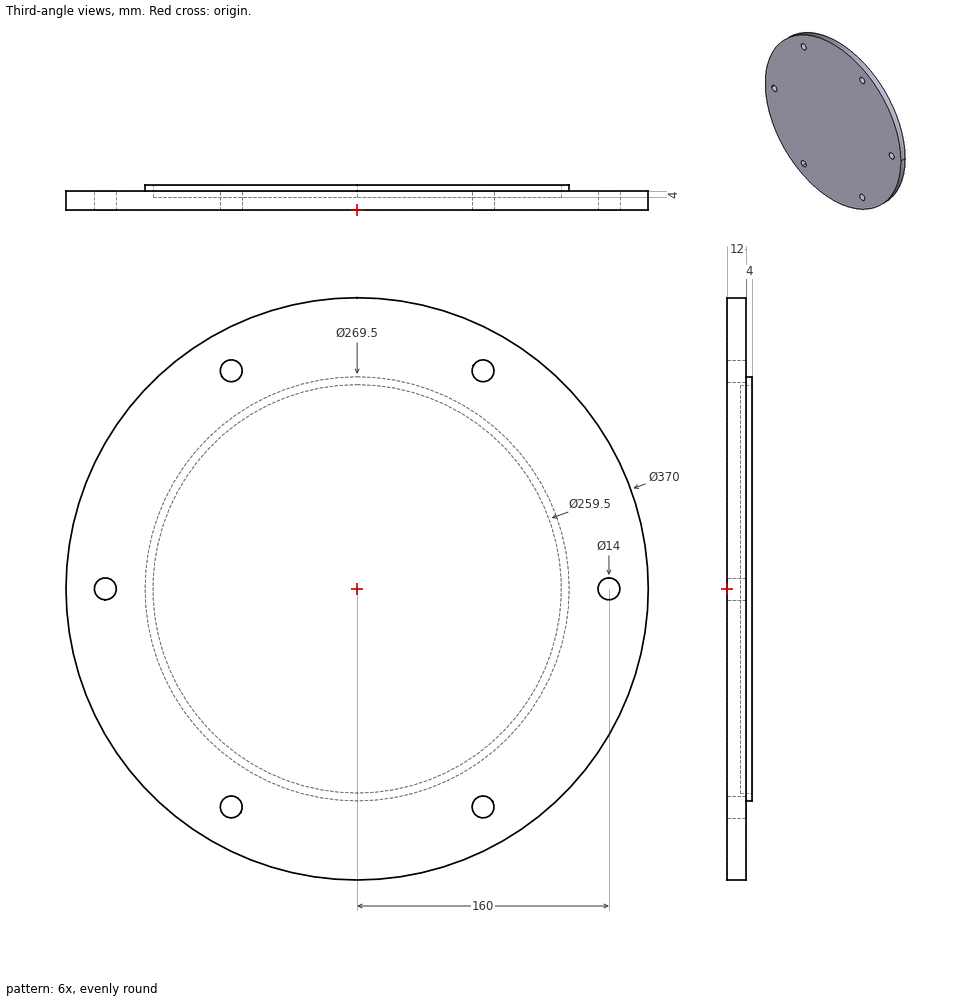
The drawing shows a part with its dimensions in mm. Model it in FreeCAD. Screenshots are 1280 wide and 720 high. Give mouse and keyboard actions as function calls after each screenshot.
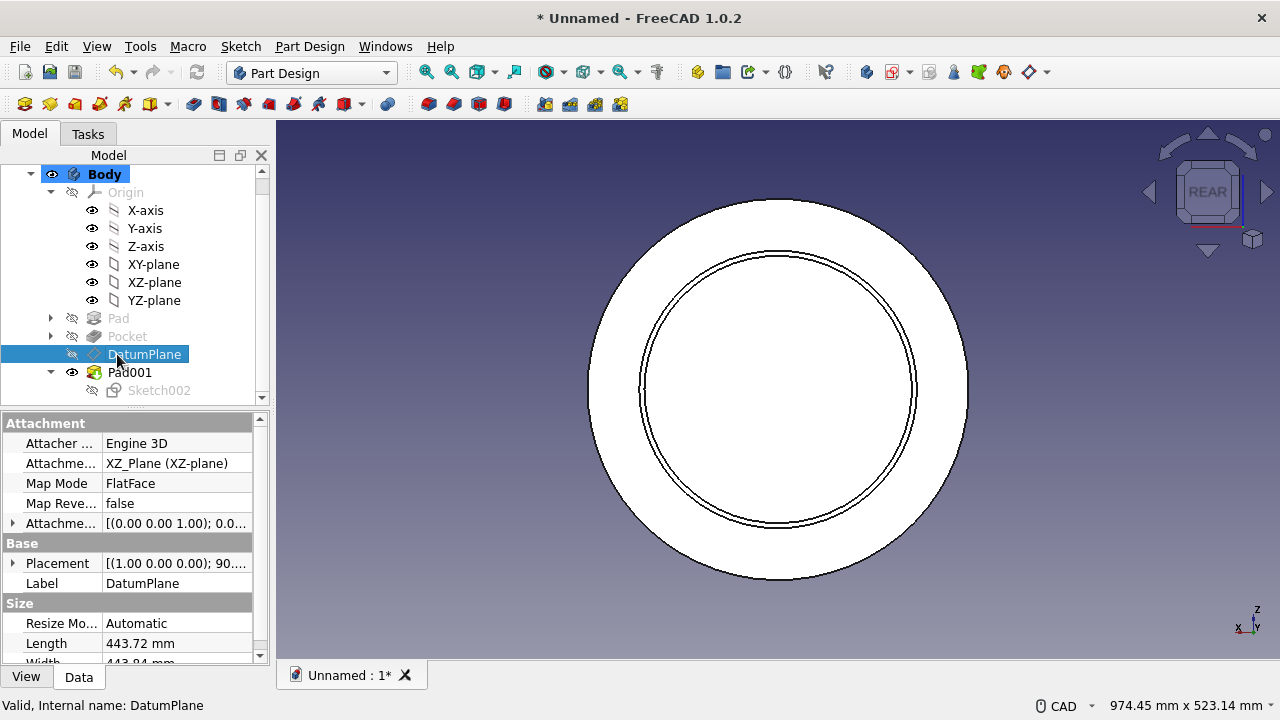
click(778, 552)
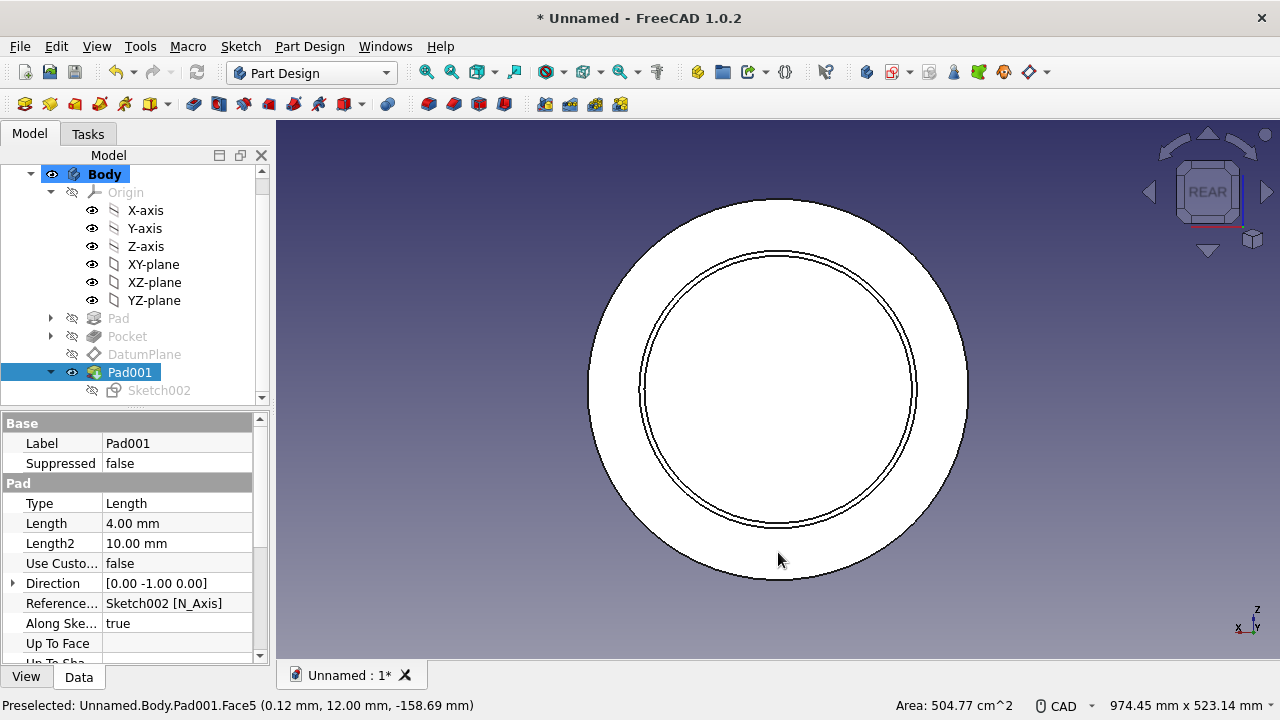
click(892, 72)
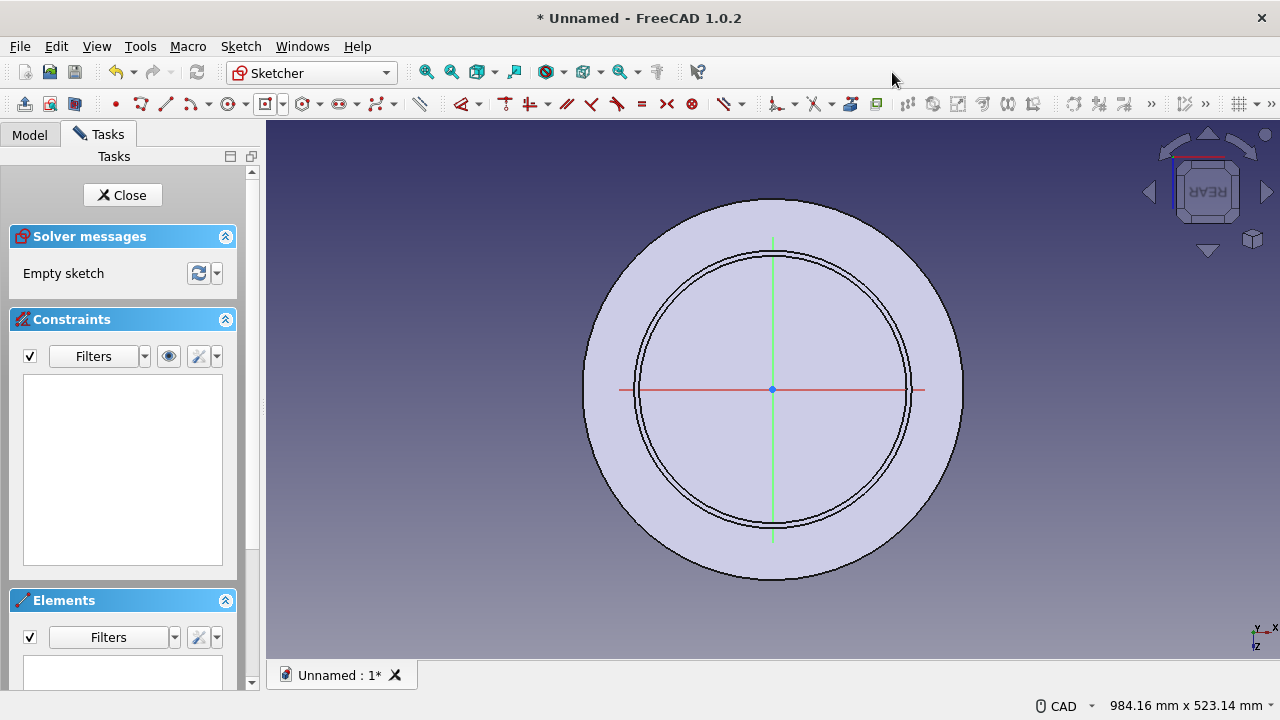
click(75, 104)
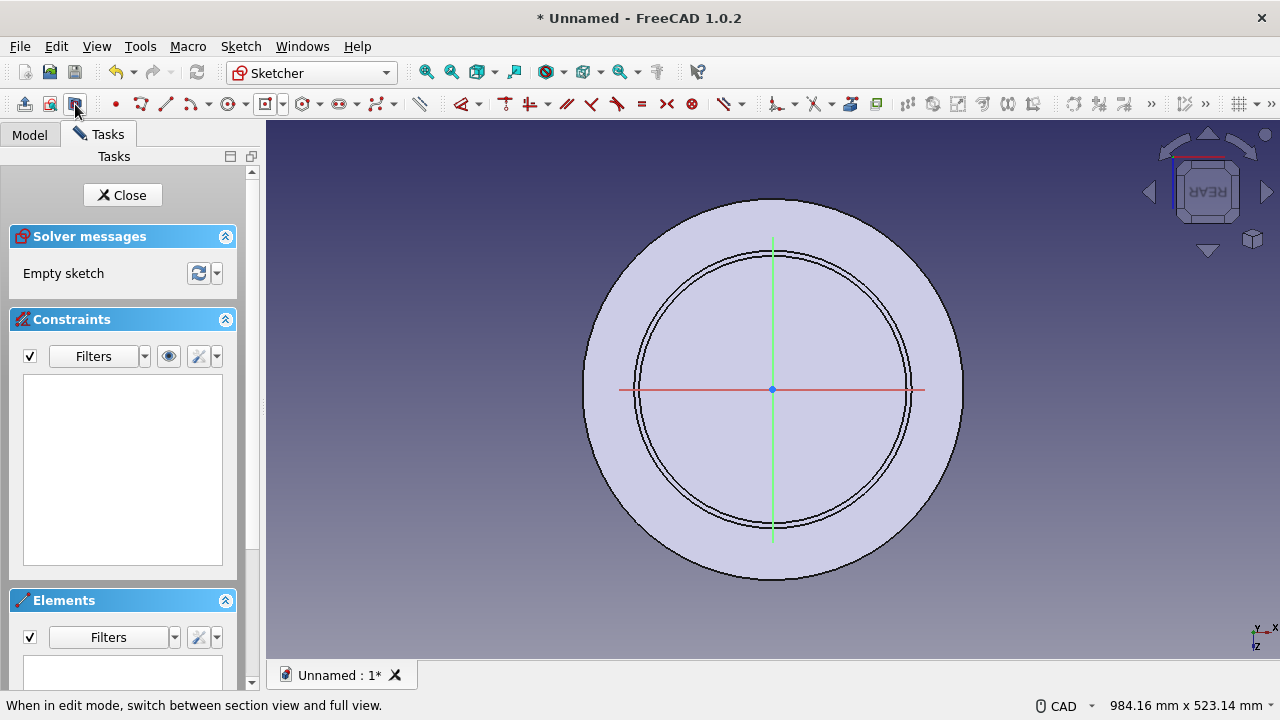
scroll(950, 389, up, 15)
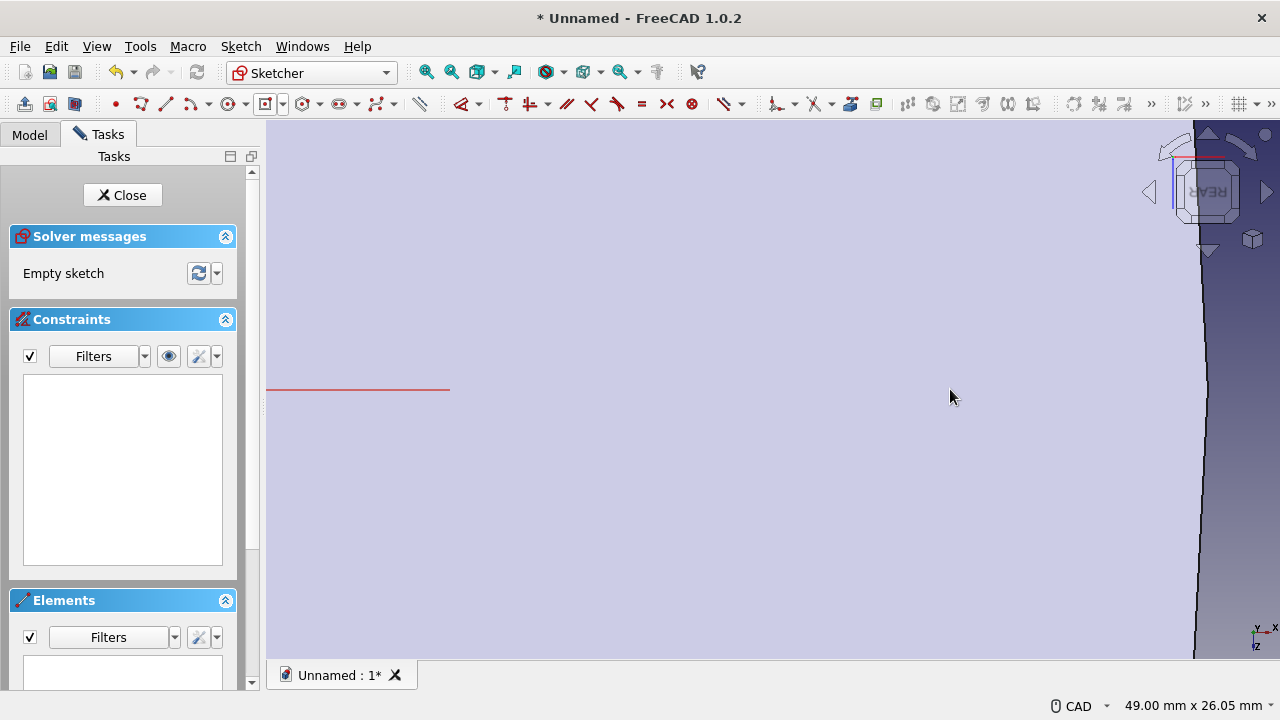
click(228, 104)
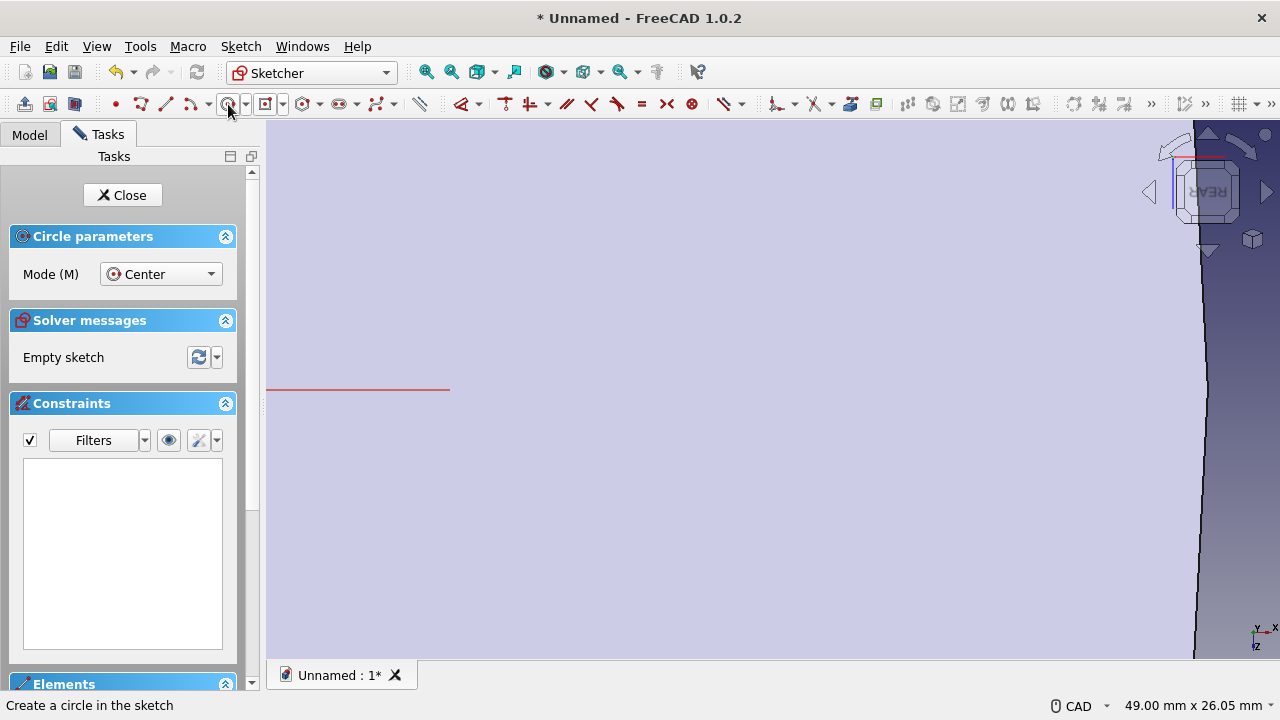
click(691, 389)
click(793, 287)
key(Escape)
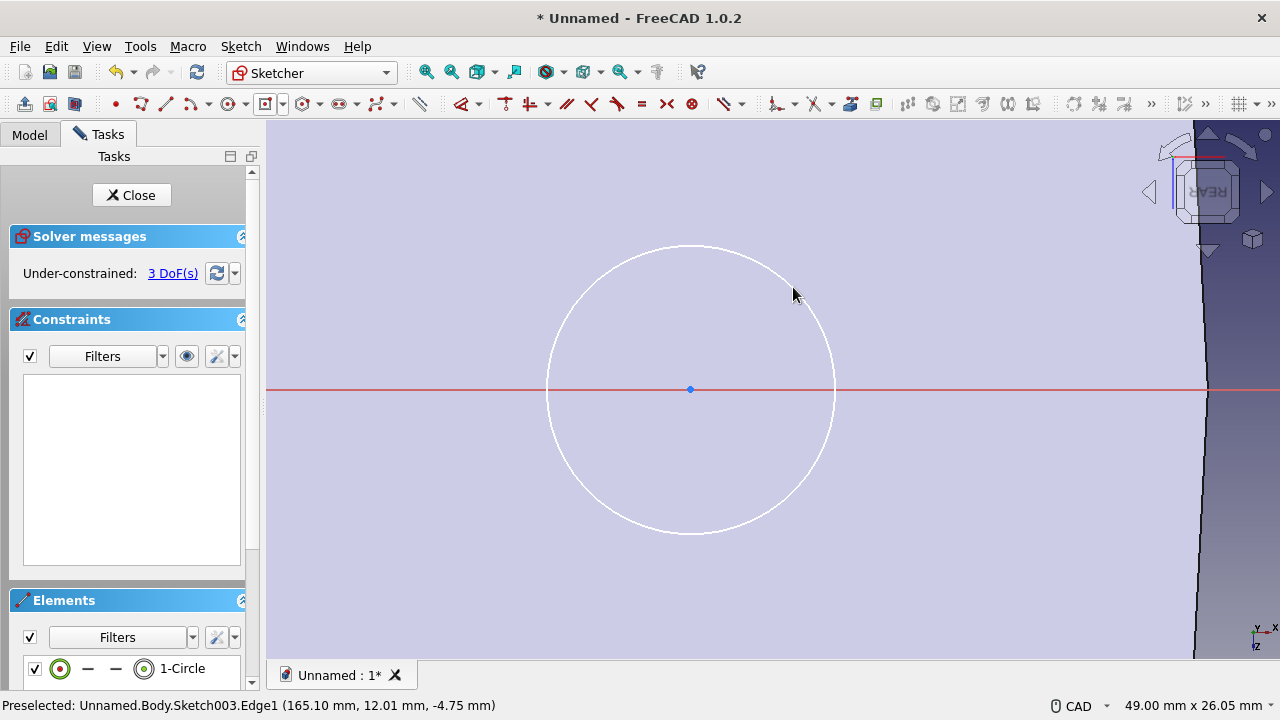
click(691, 390)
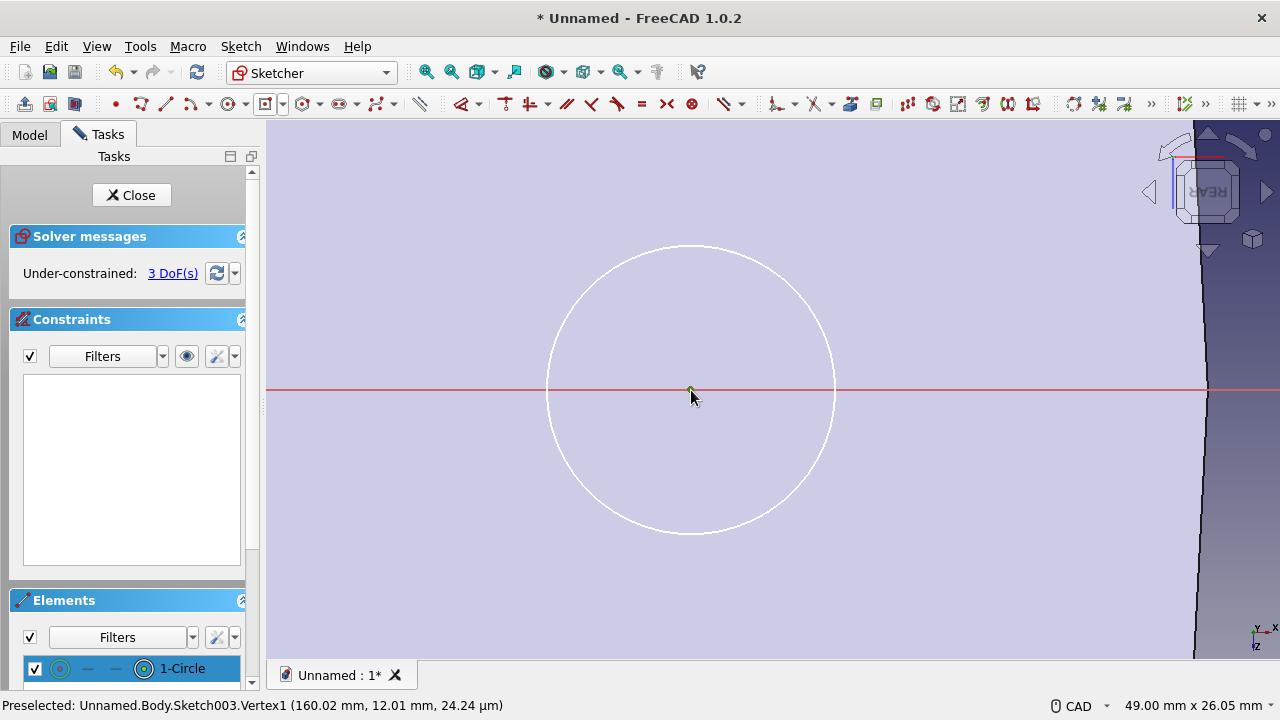
click(353, 389)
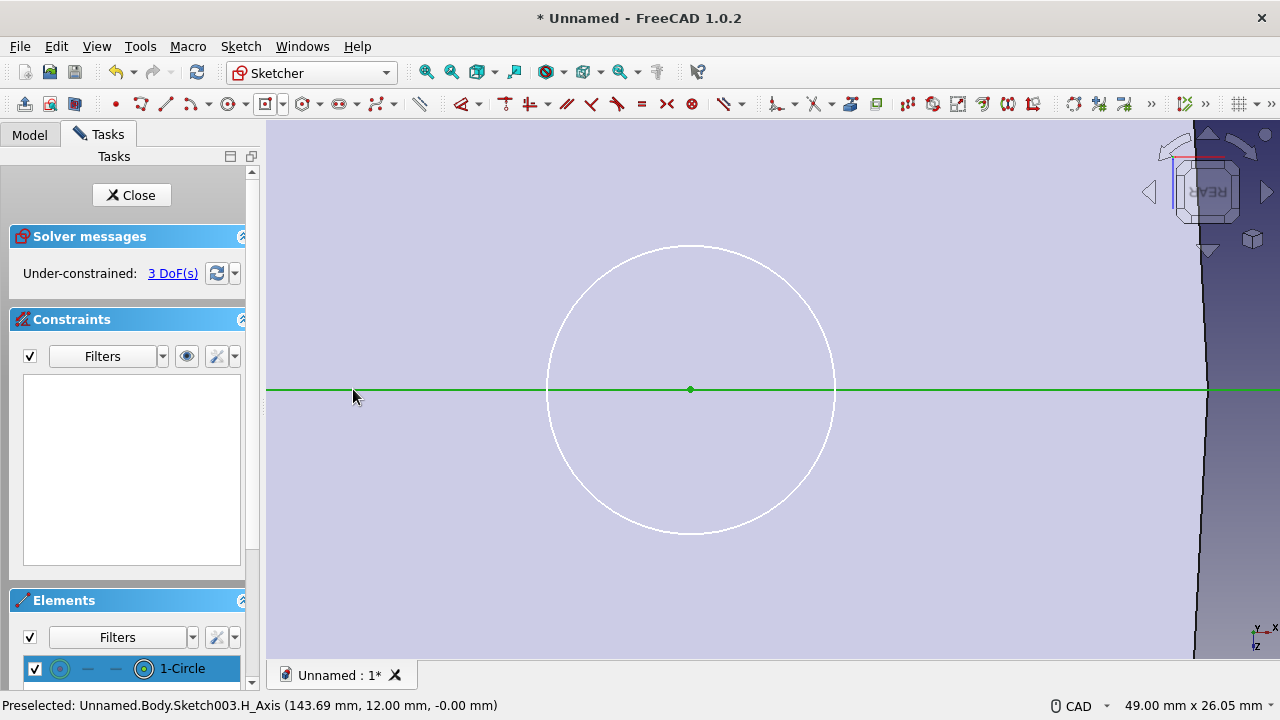
click(505, 104)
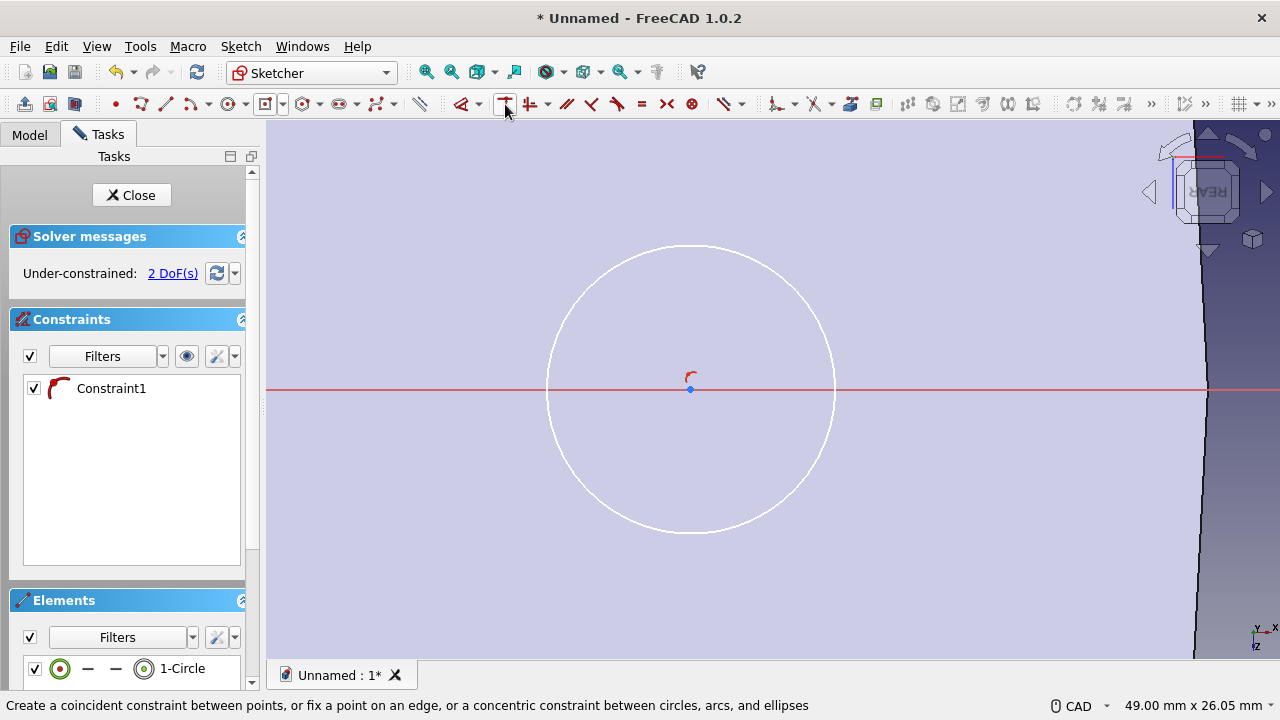
click(460, 104)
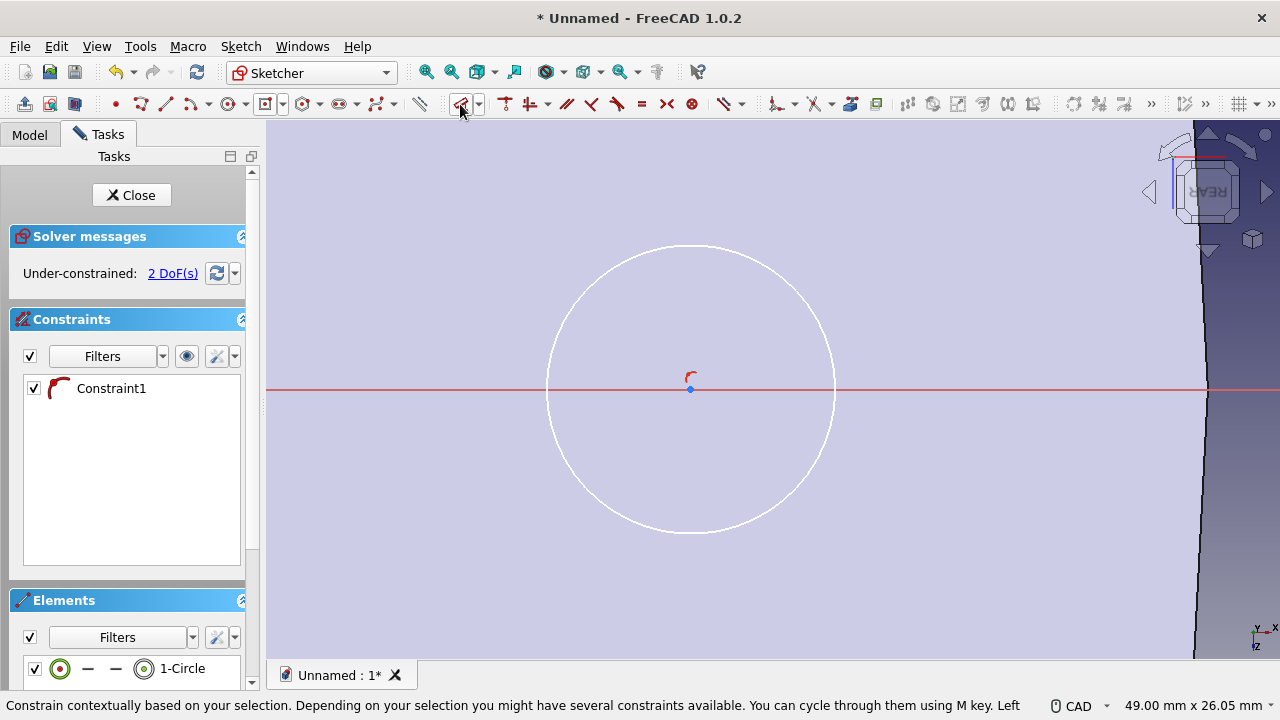
click(793, 287)
click(816, 264)